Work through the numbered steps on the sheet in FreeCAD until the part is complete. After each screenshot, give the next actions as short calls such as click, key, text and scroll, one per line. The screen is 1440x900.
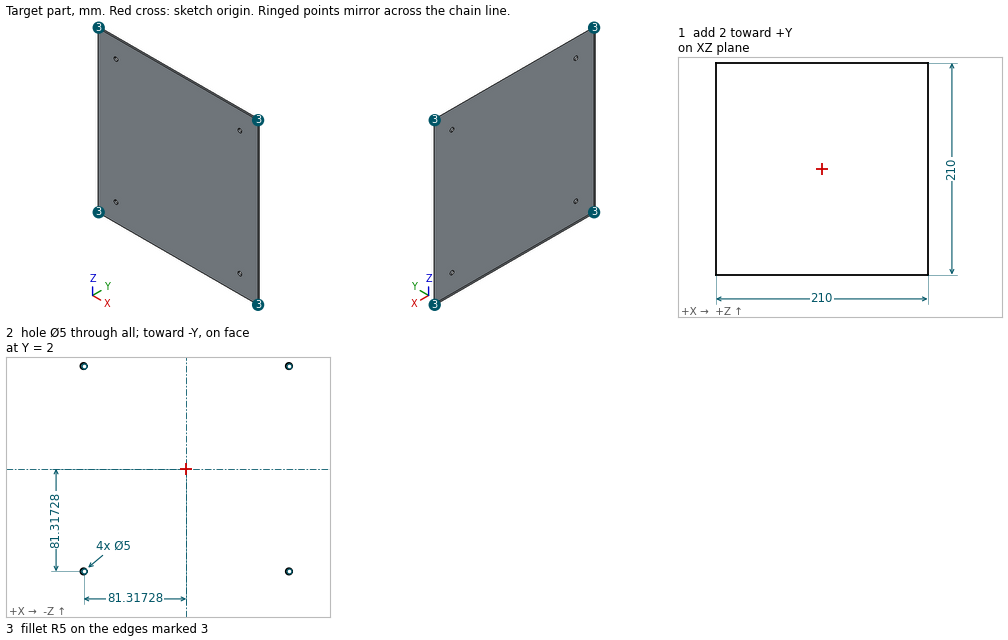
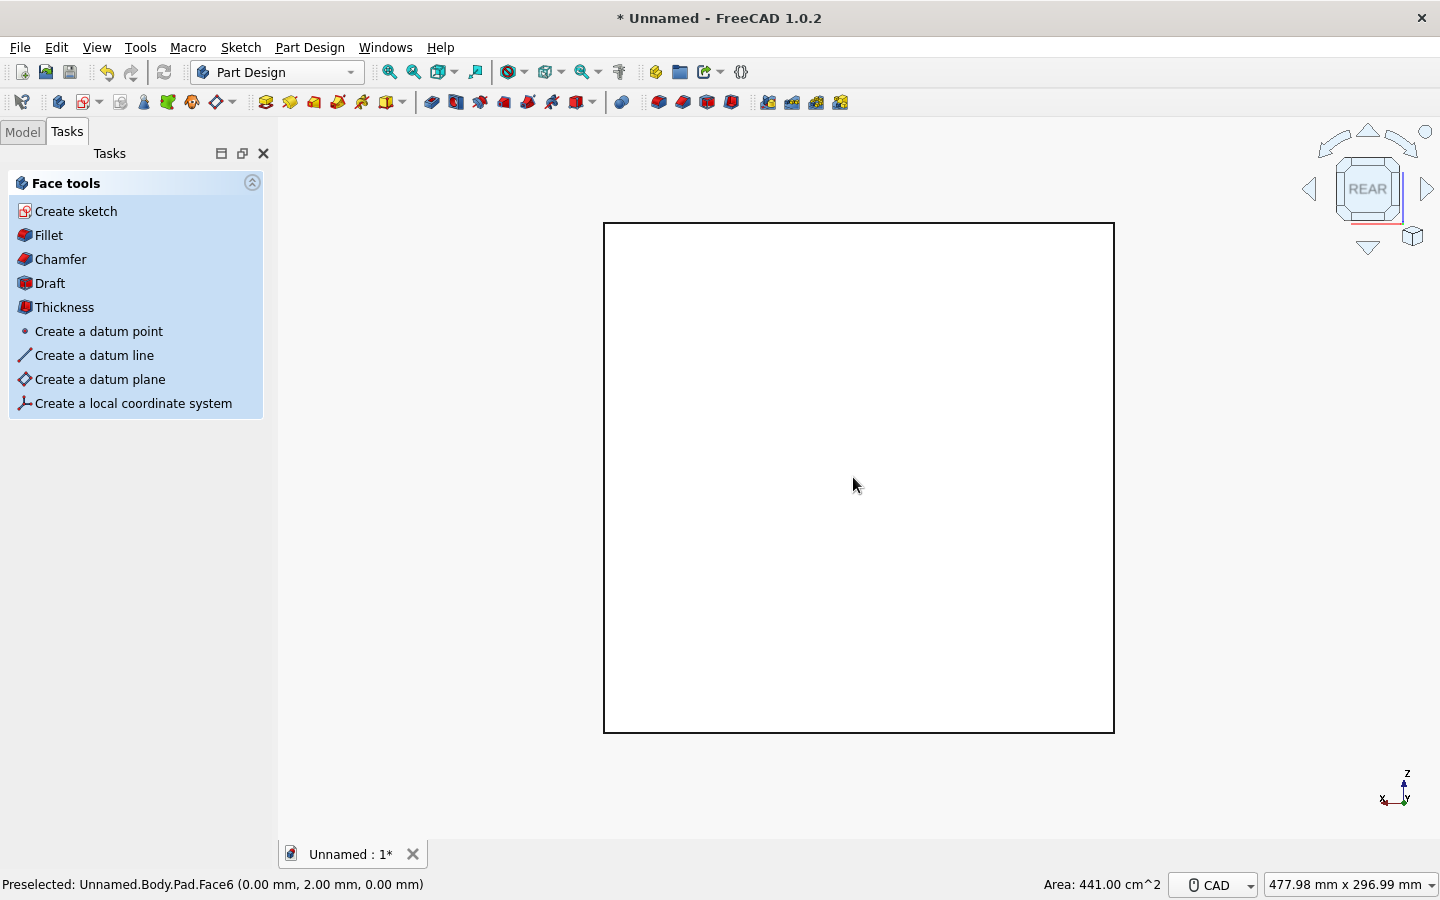
click(84, 102)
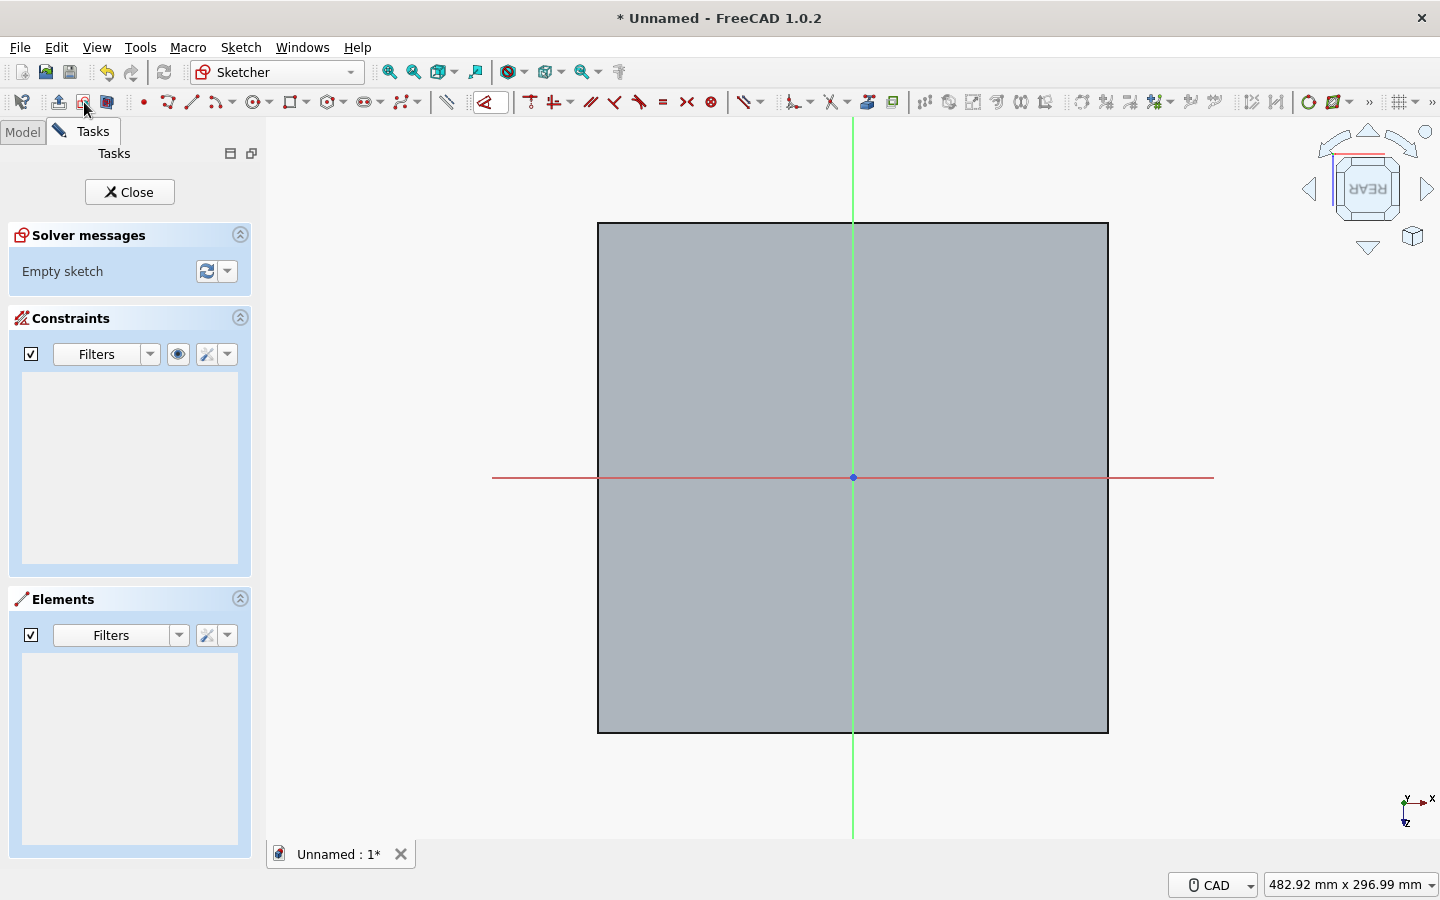
click(254, 102)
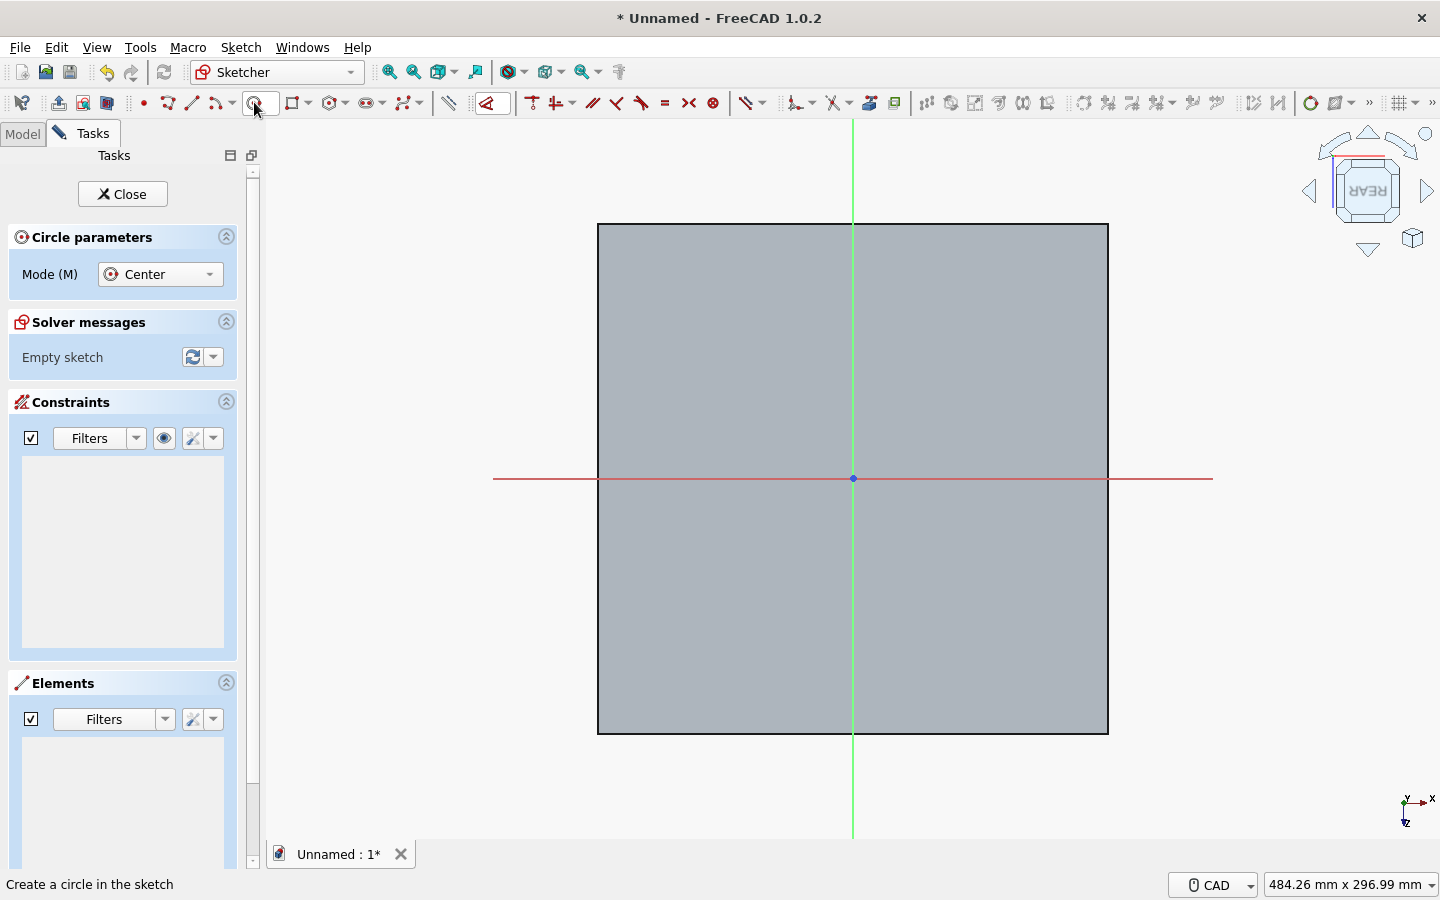
scroll(656, 676, up, 7)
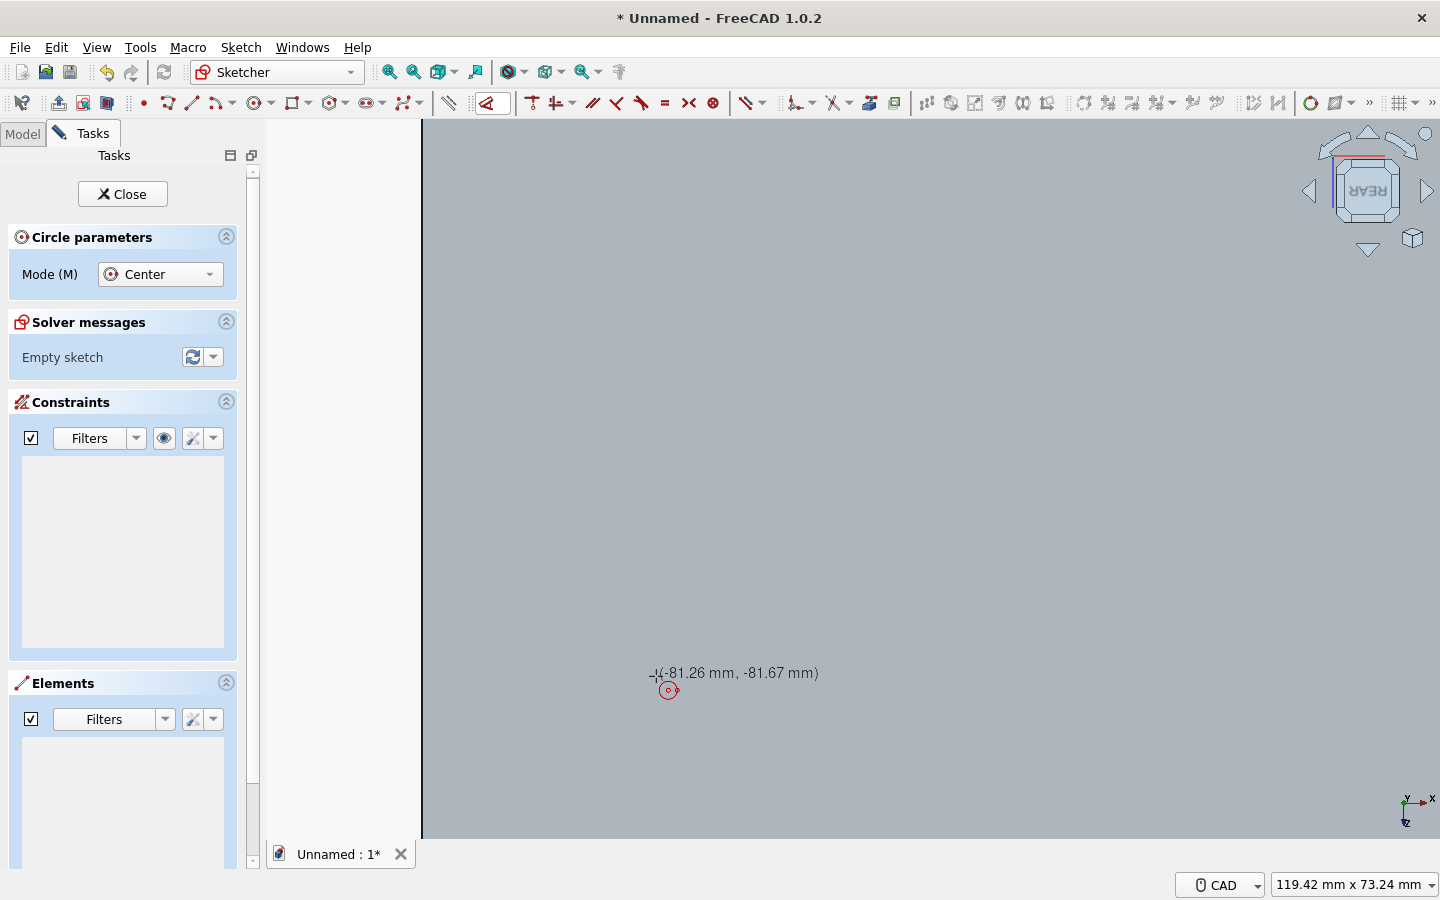
scroll(496, 739, down, 6)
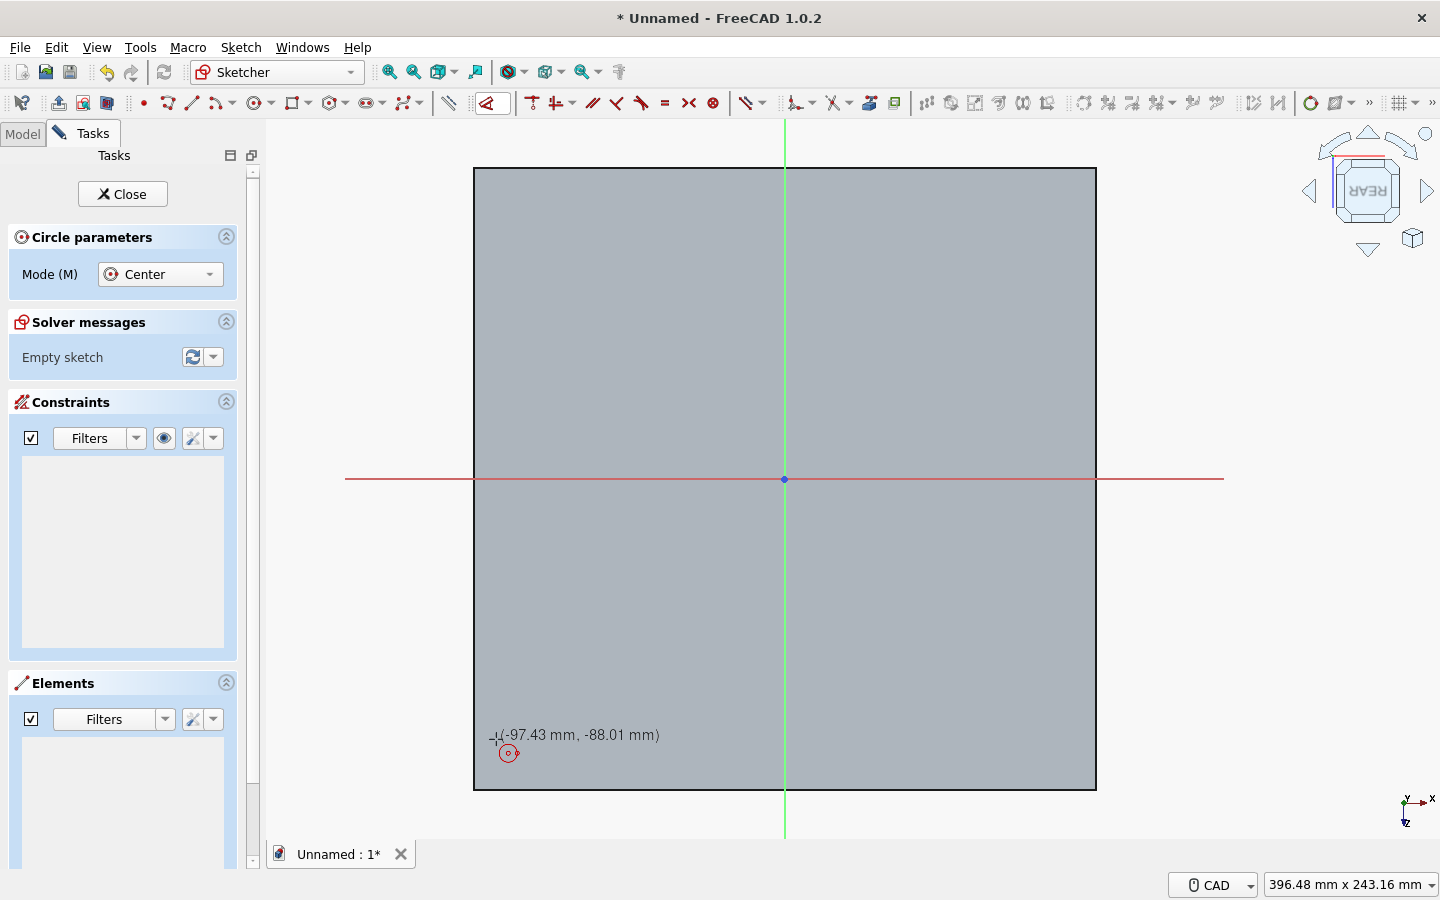
click(544, 720)
move(549, 715)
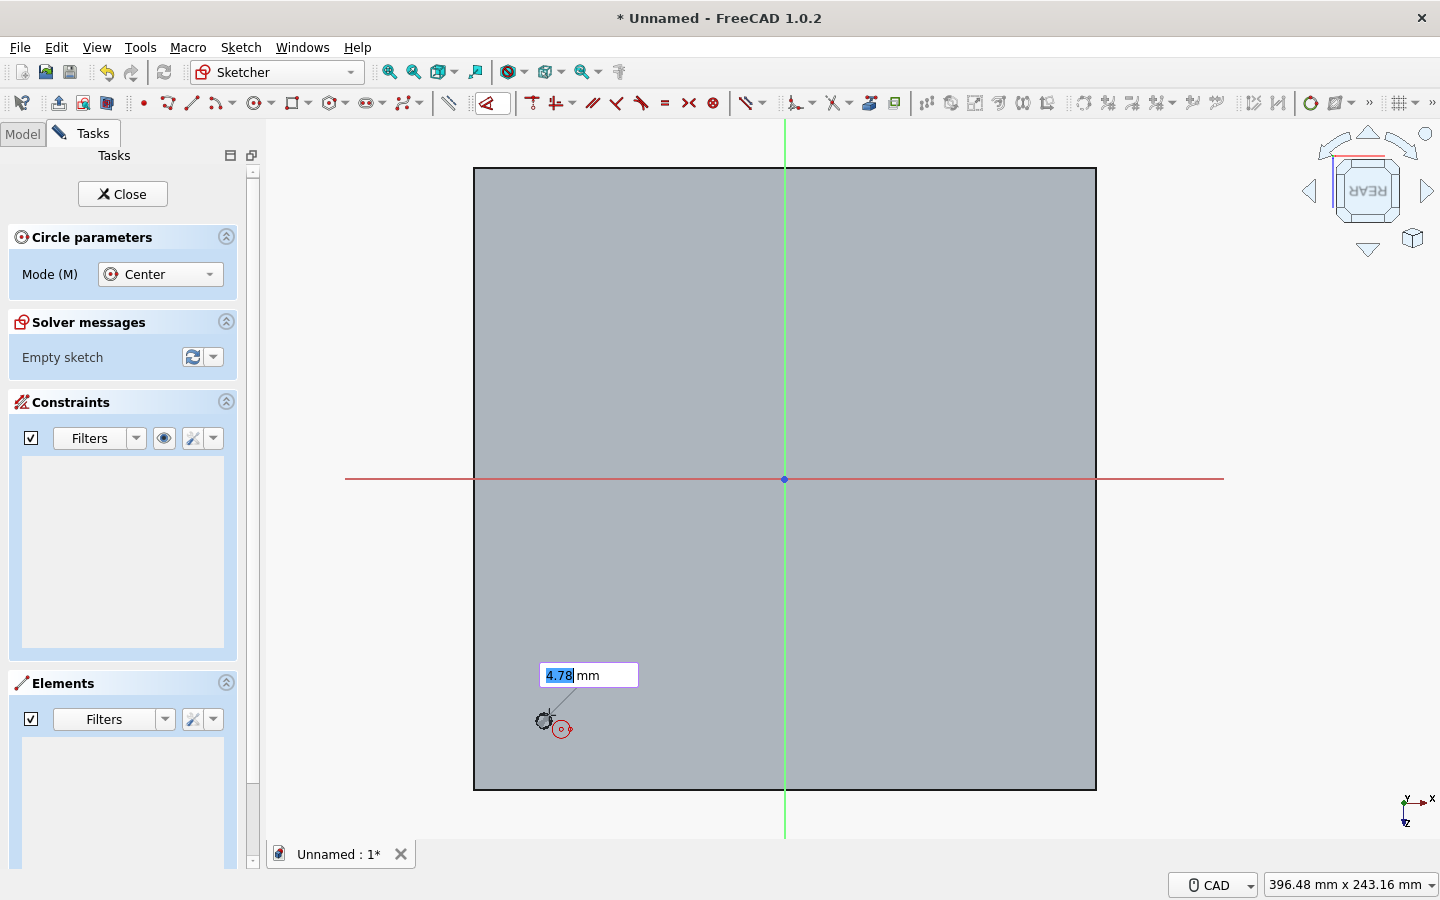
text(5)
key(Return)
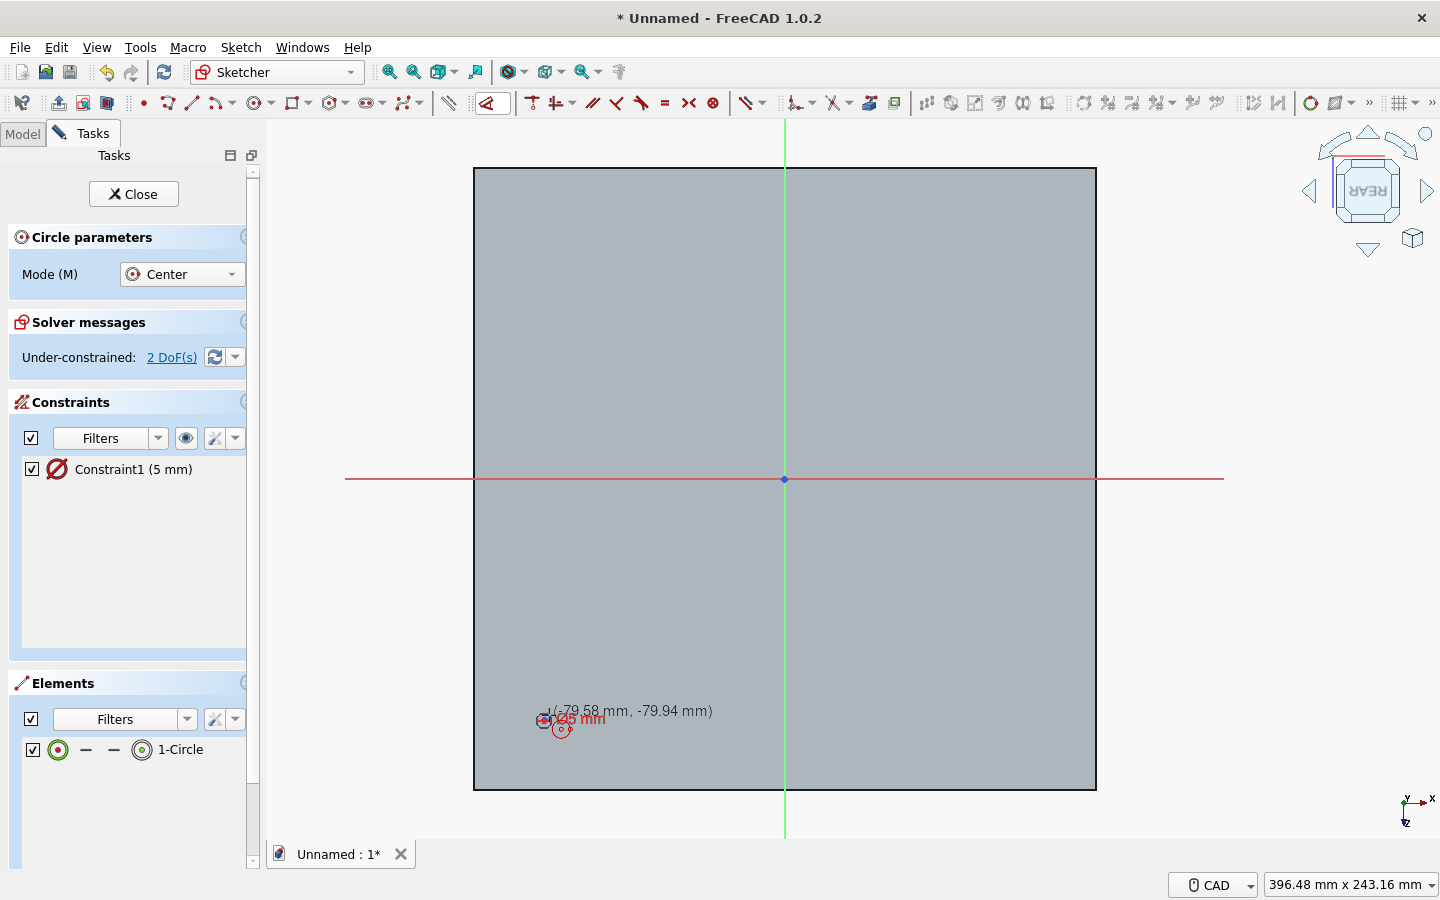
scroll(544, 239, up, 6)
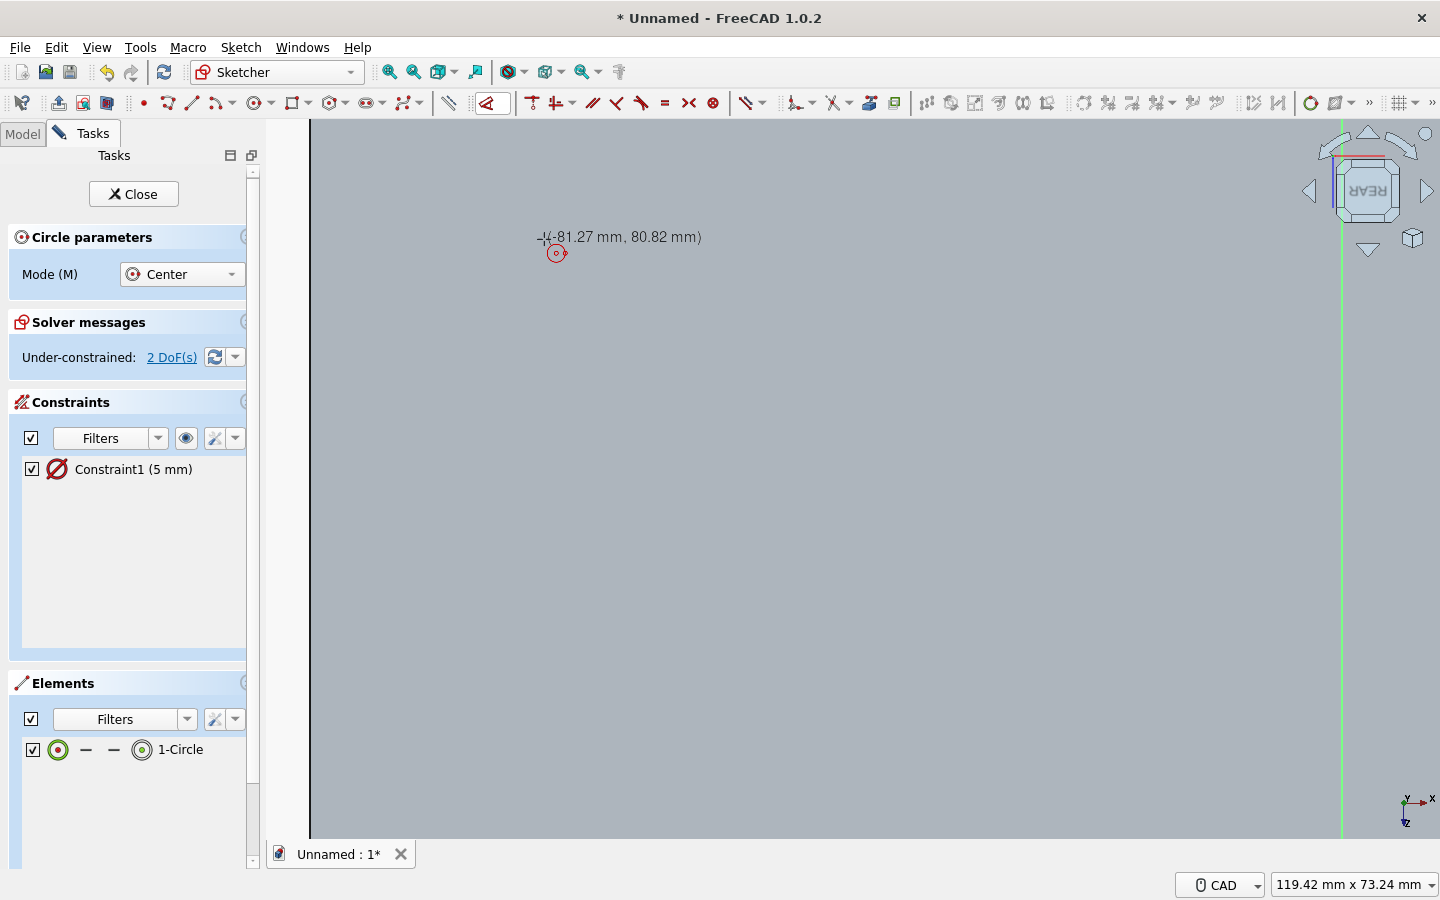
scroll(544, 239, down, 6)